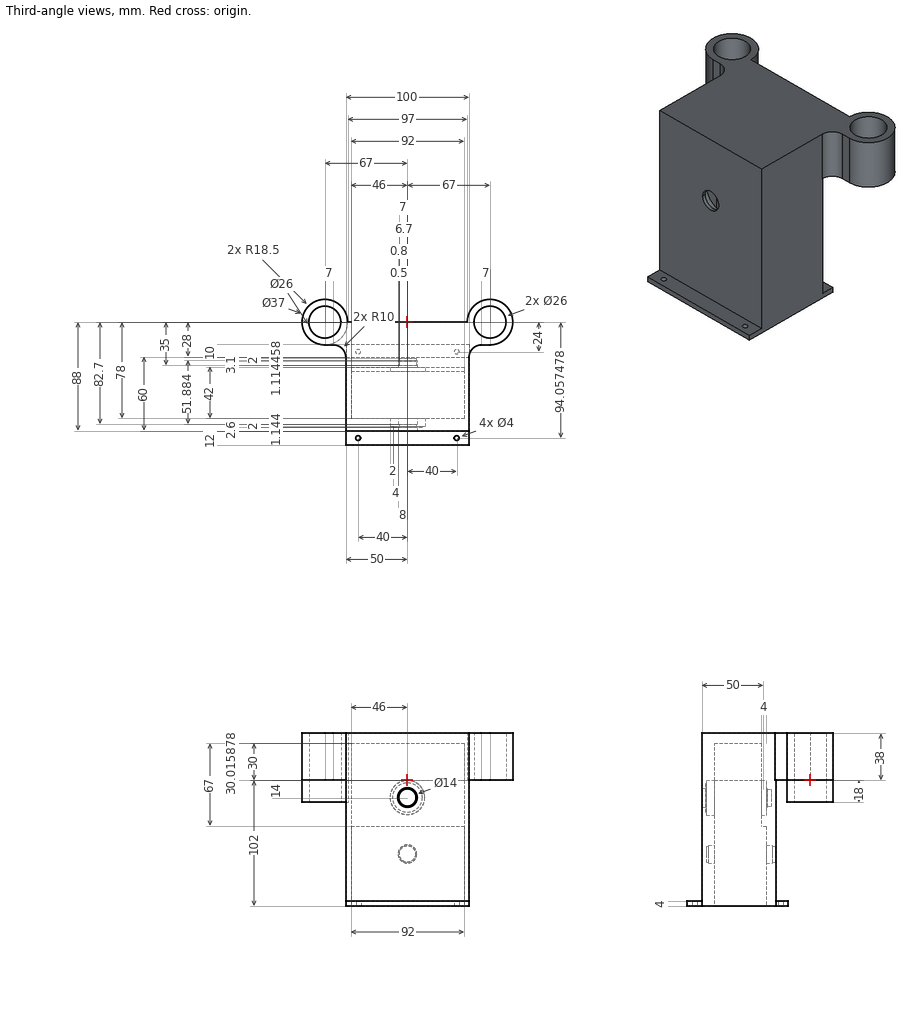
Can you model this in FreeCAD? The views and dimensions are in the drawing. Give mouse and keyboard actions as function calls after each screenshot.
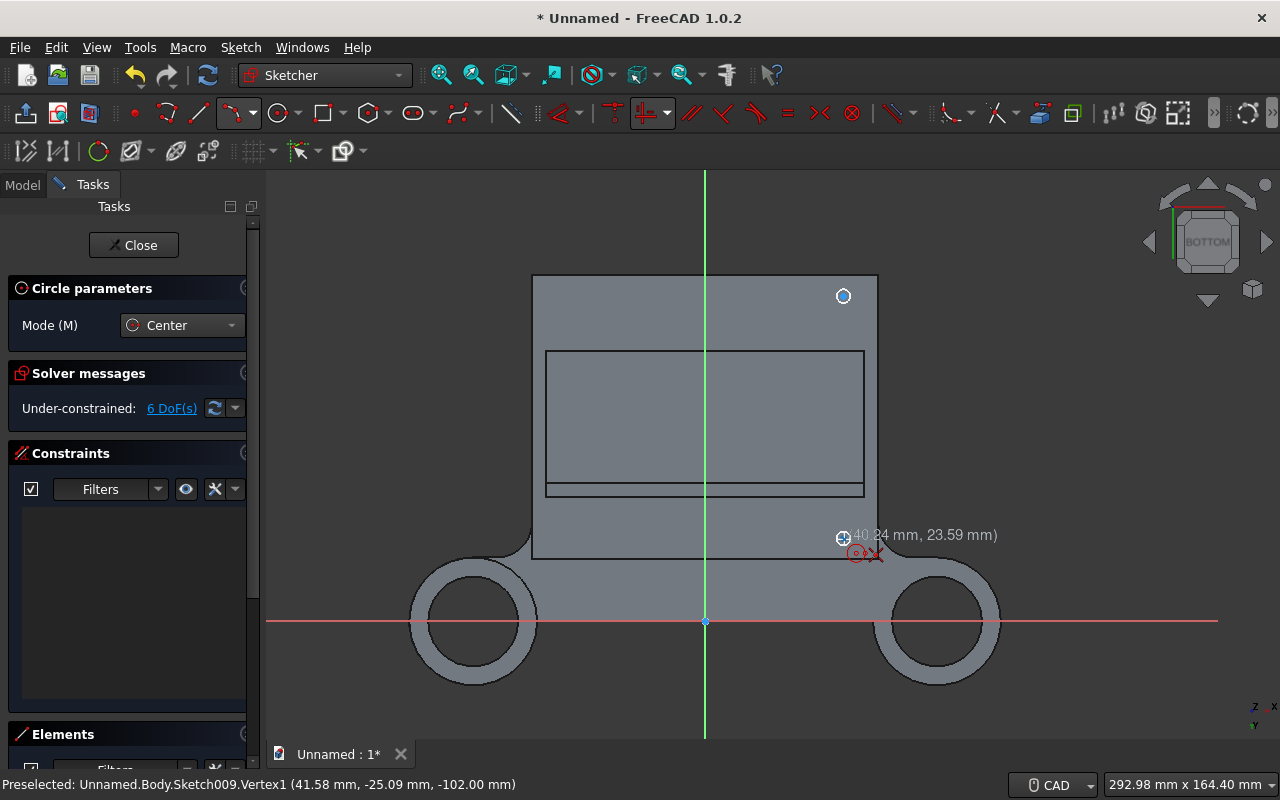
scroll(567, 296, up, 6)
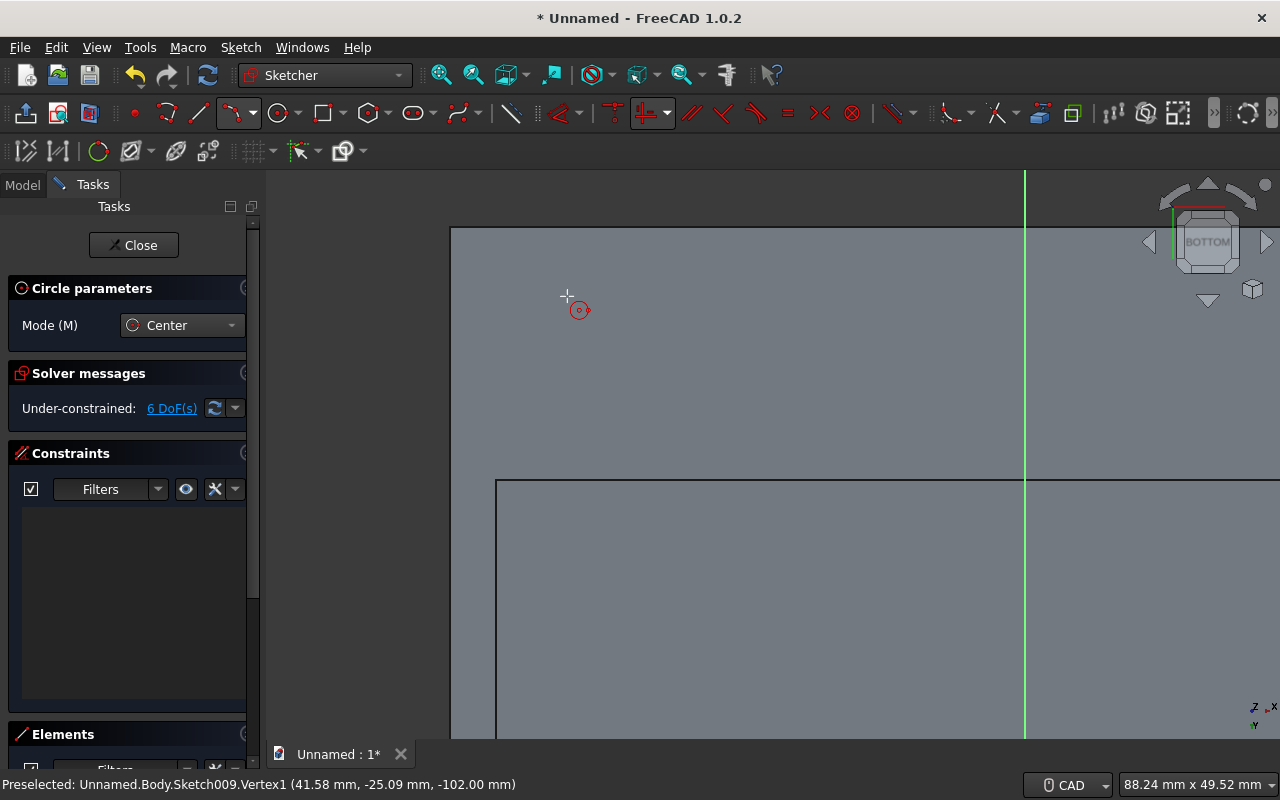
click(565, 295)
click(581, 279)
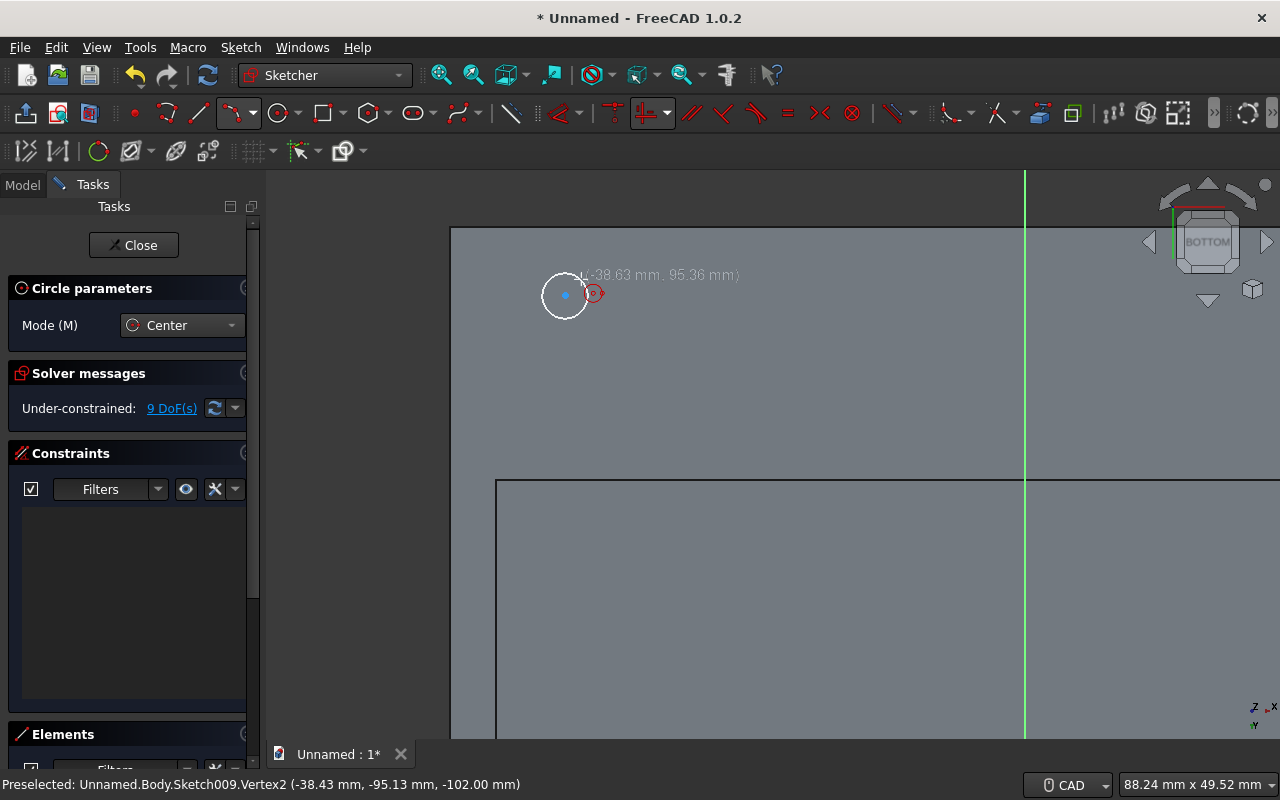
scroll(566, 295, down, 6)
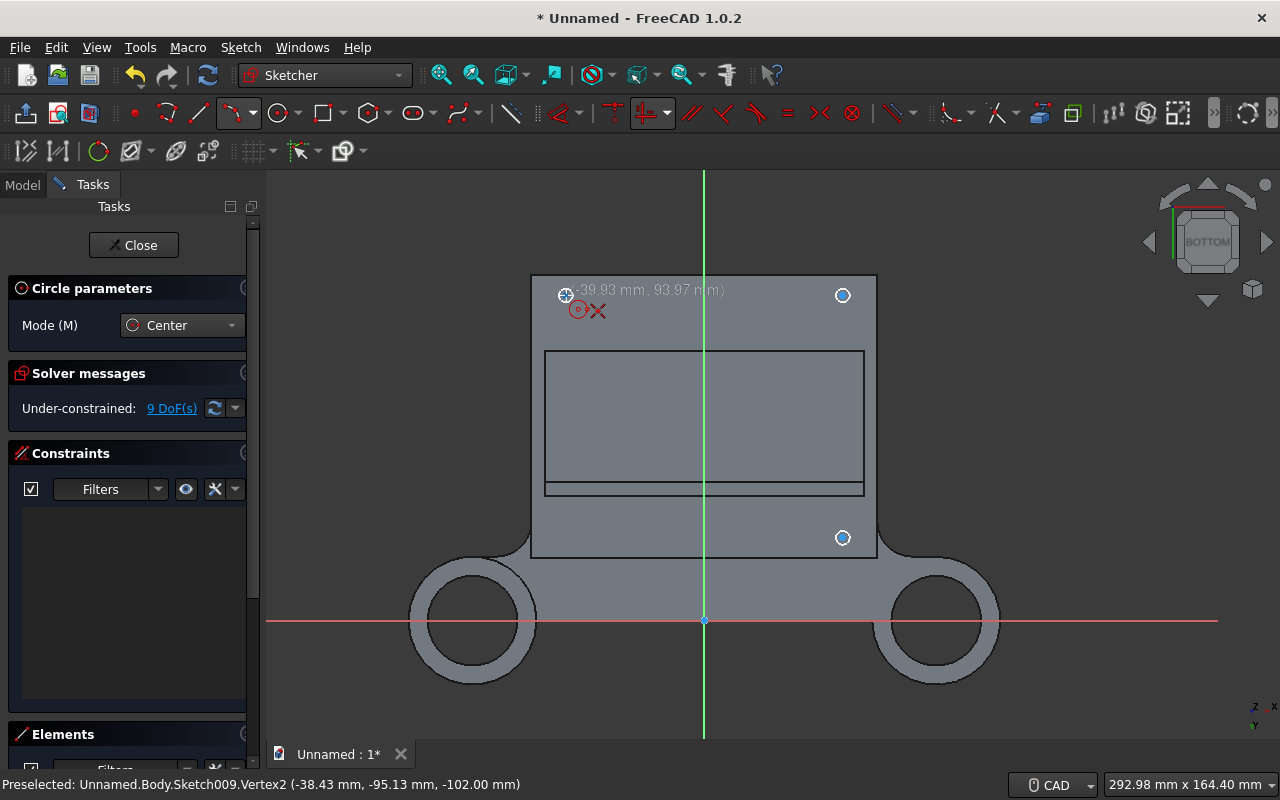
scroll(566, 538, up, 6)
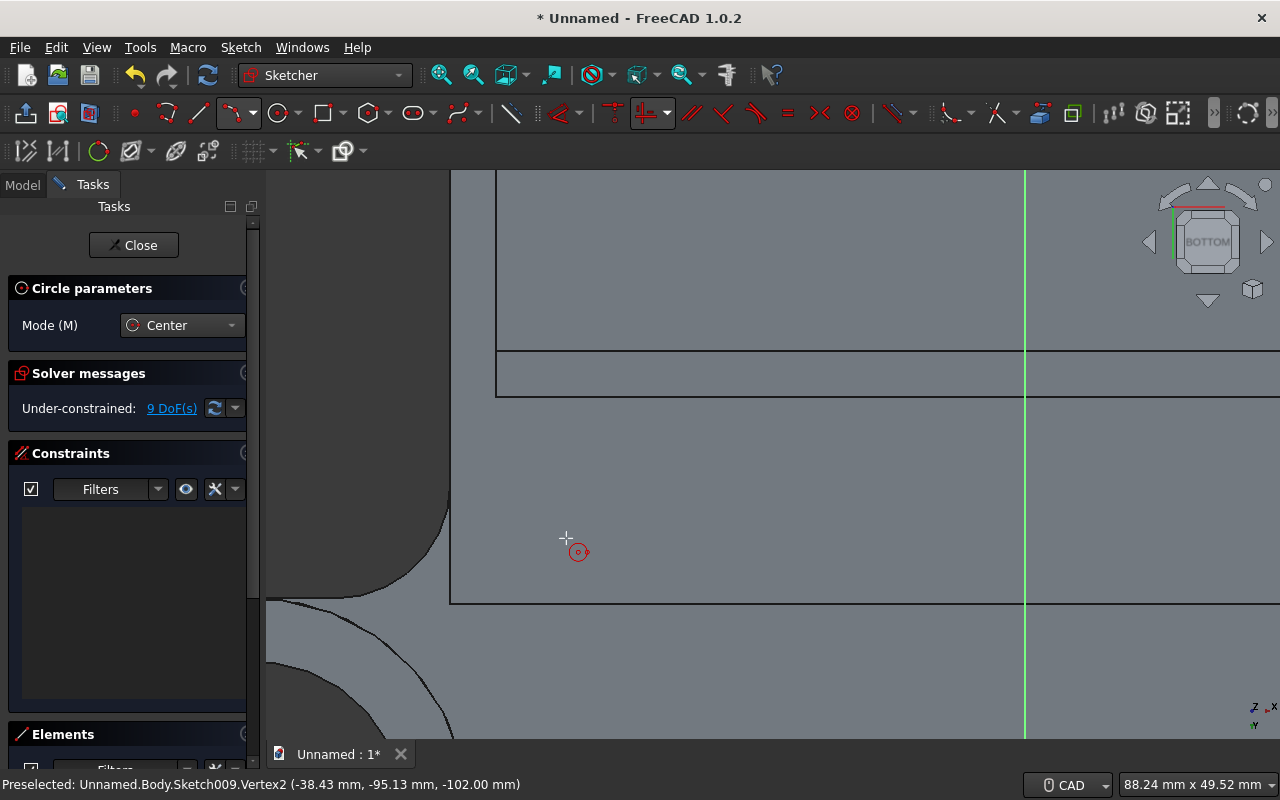
click(565, 535)
click(581, 519)
key(Escape)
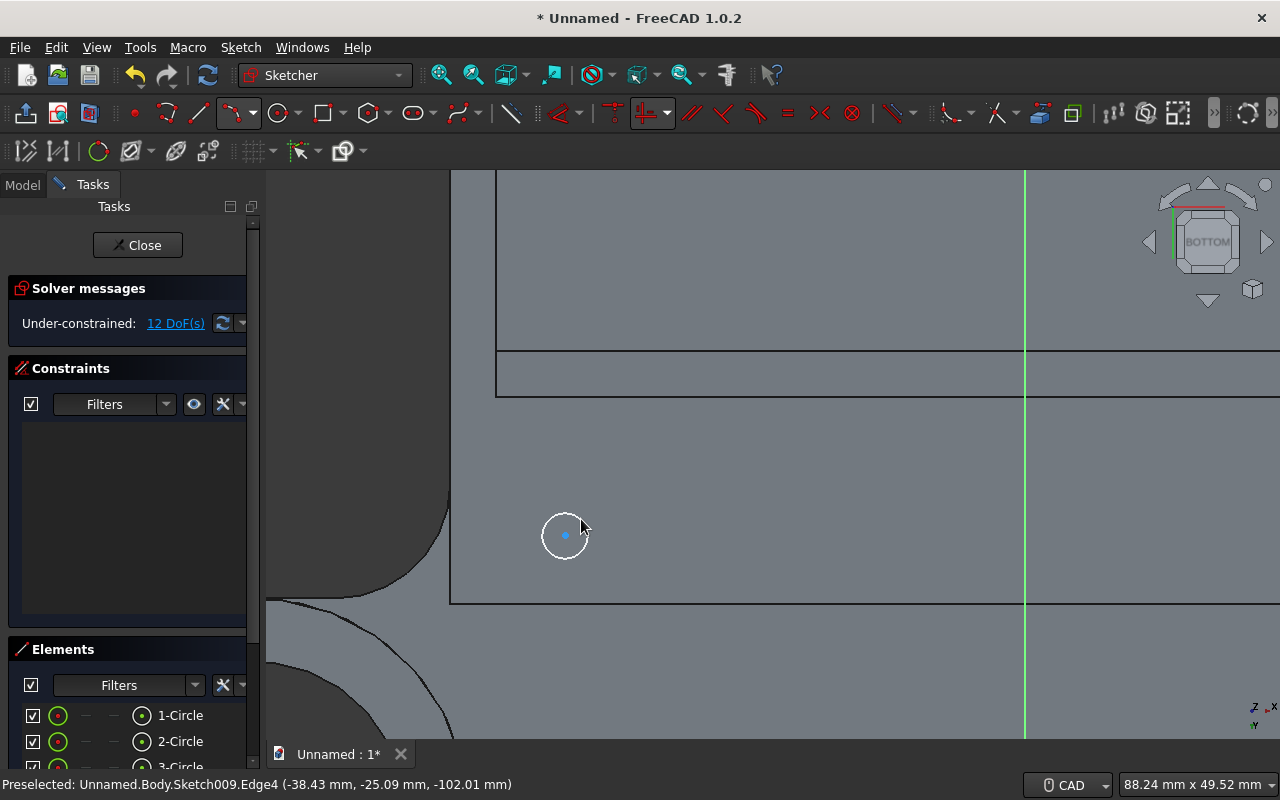
scroll(566, 539, down, 6)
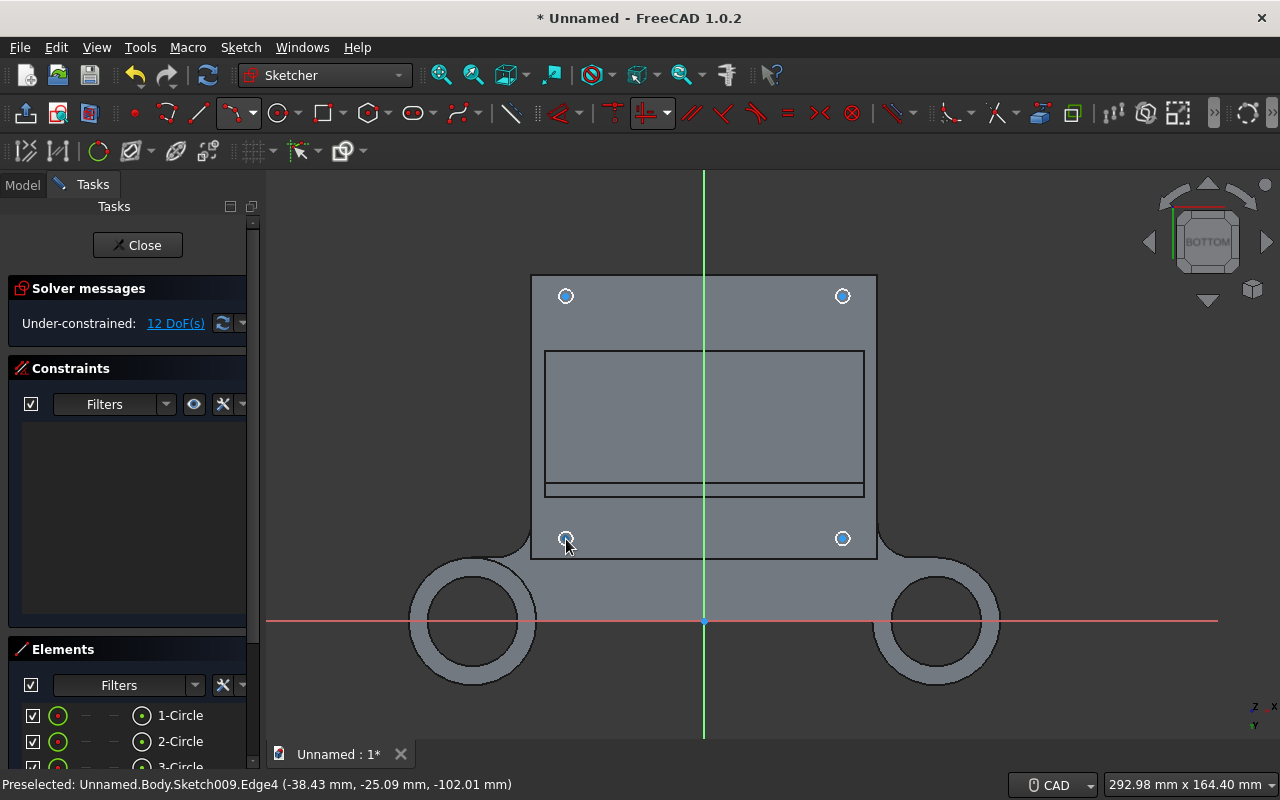
scroll(848, 291, up, 4)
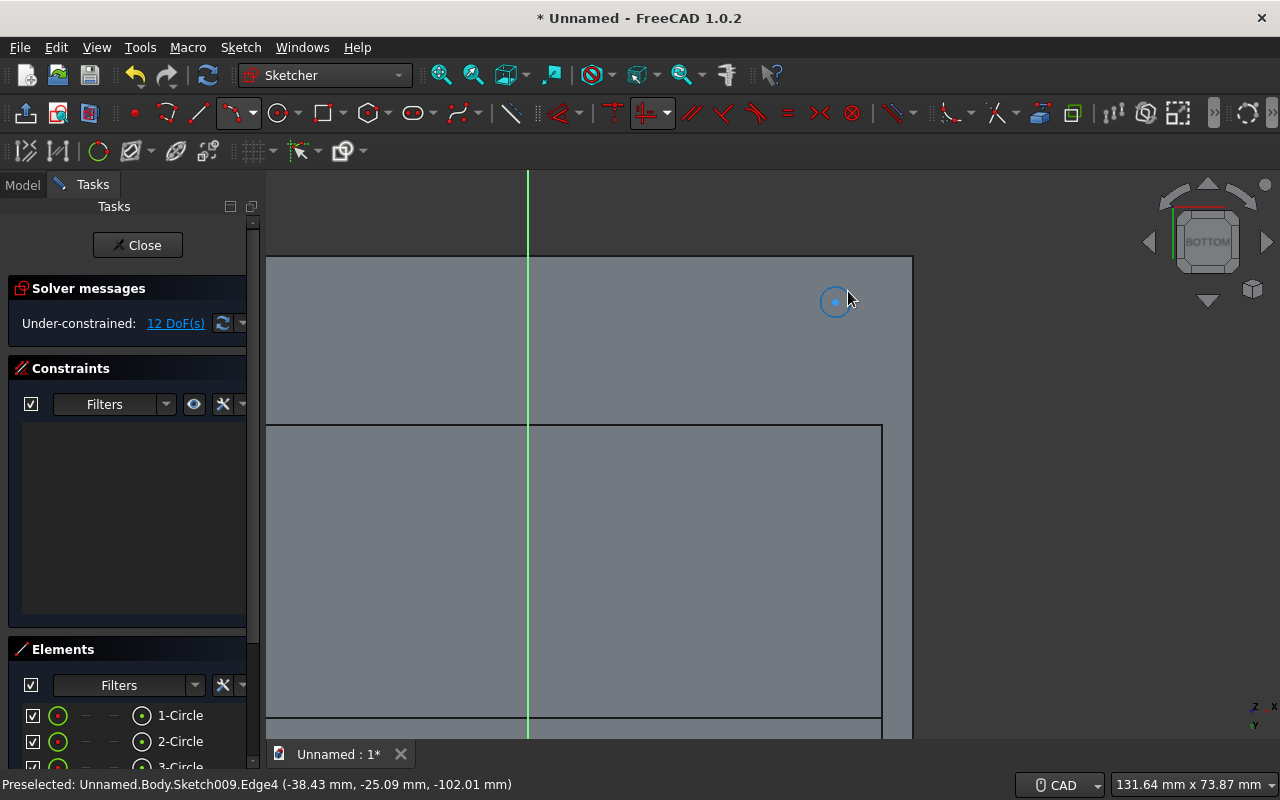
click(846, 291)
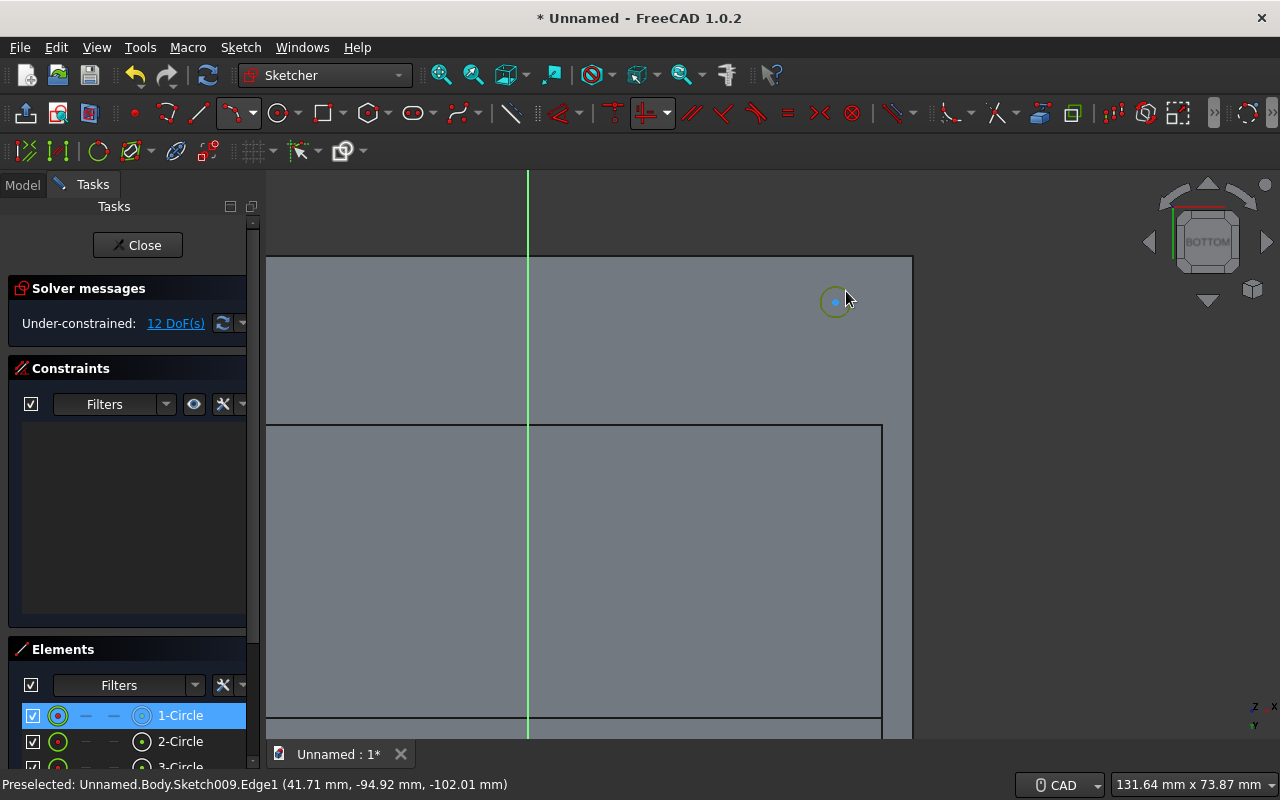
scroll(849, 290, down, 4)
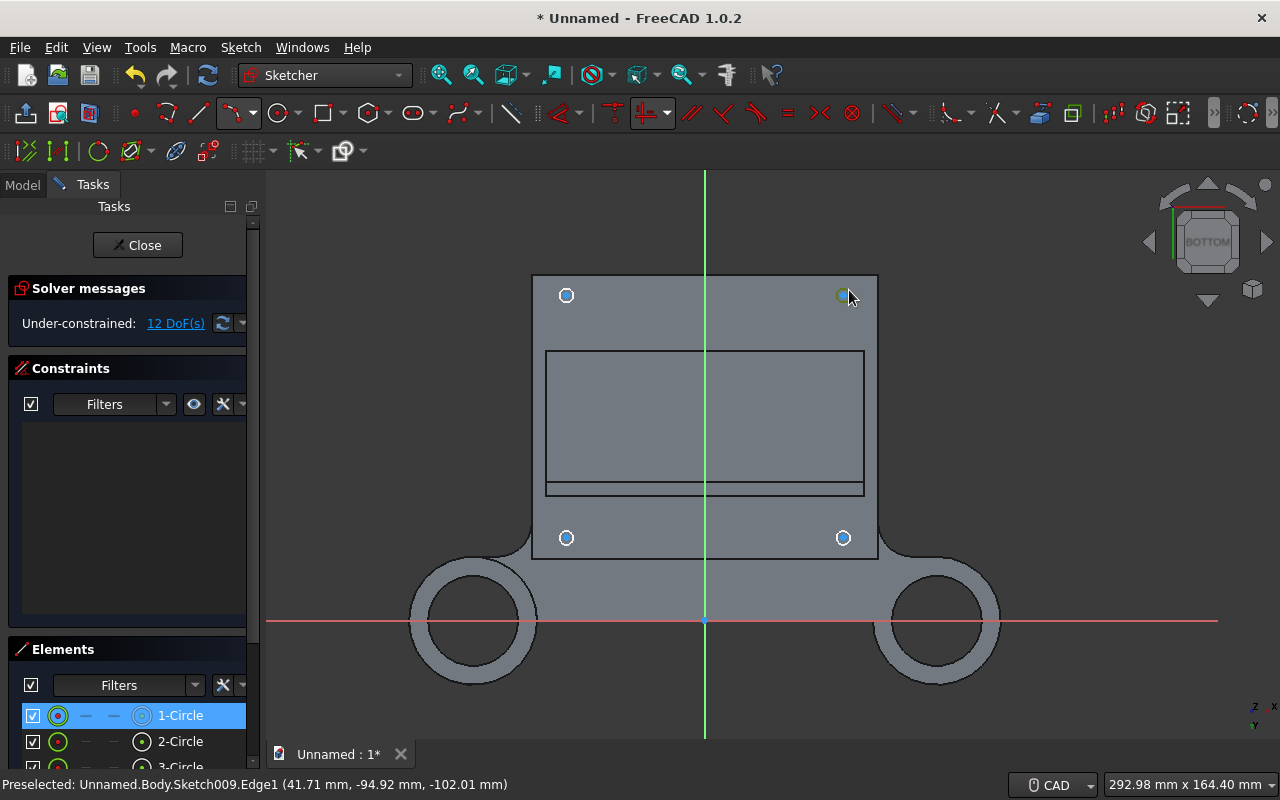
scroll(848, 533, up, 4)